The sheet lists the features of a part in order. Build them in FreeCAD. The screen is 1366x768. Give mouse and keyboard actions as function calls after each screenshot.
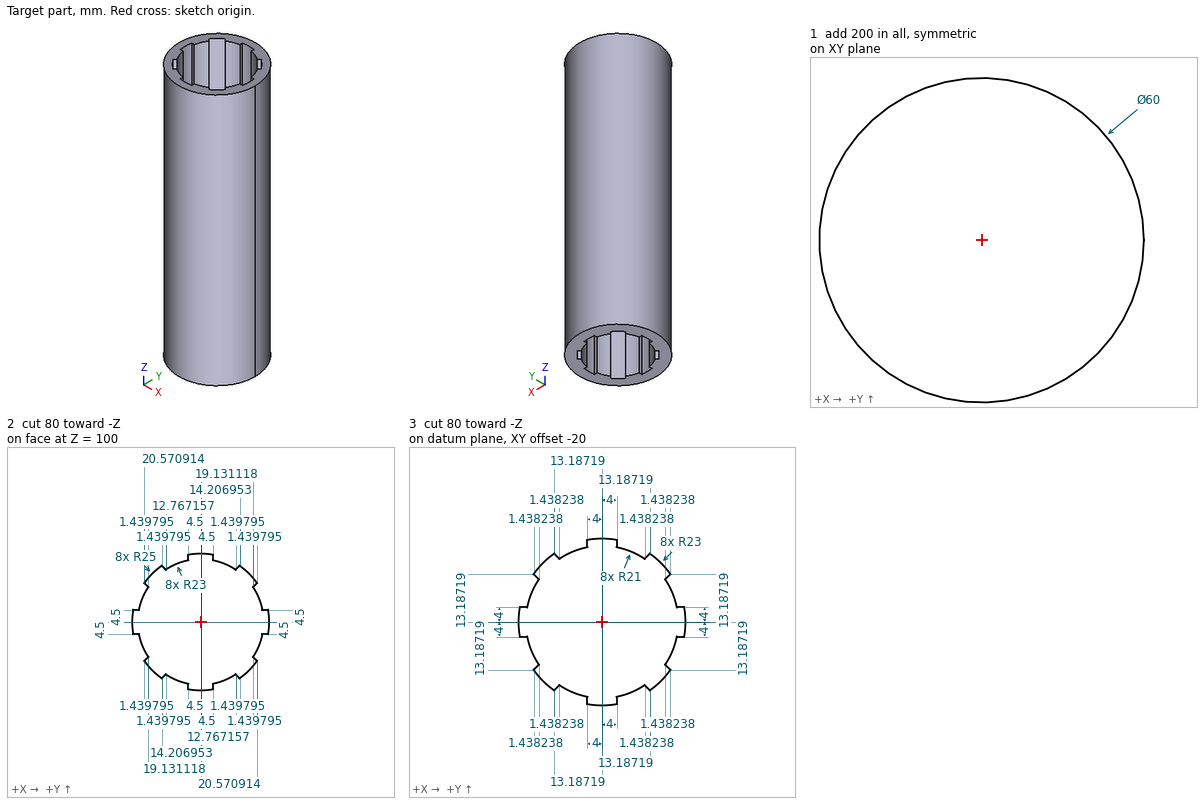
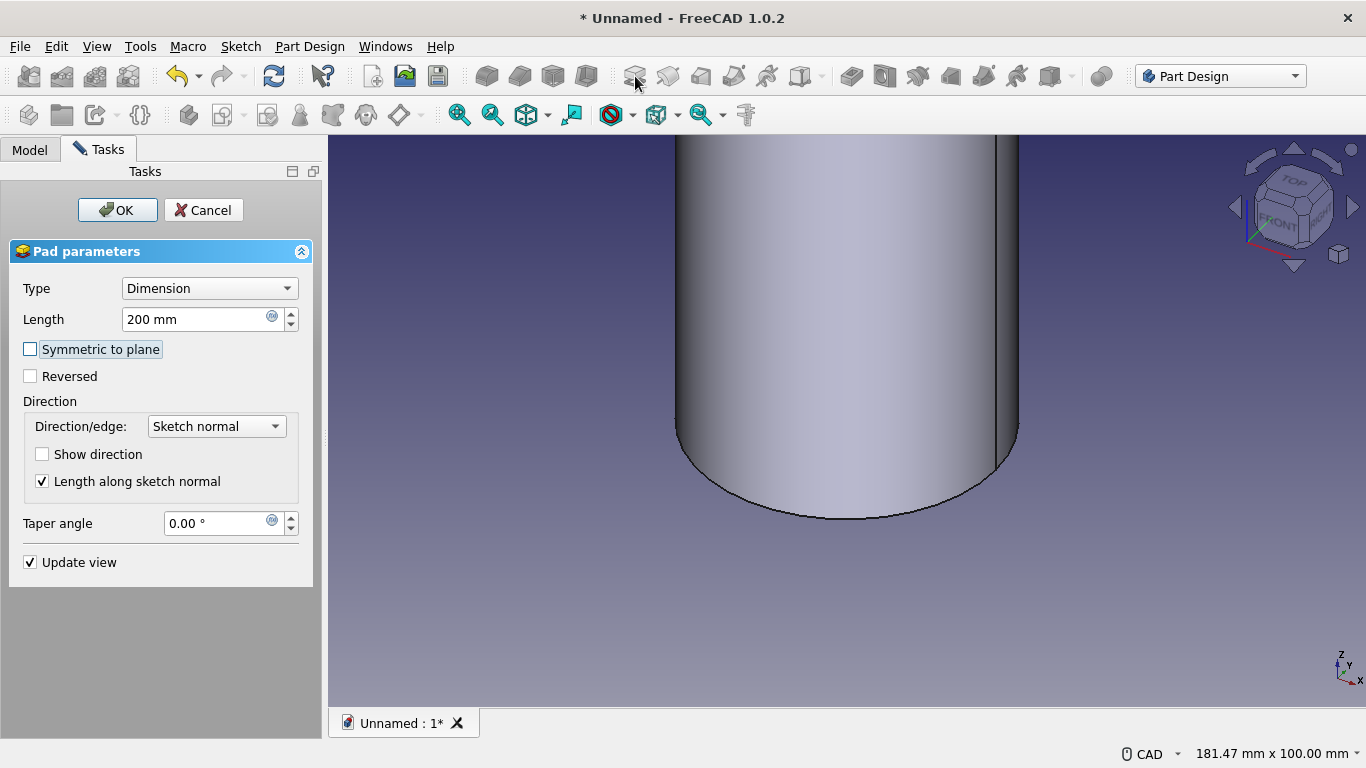
click(31, 349)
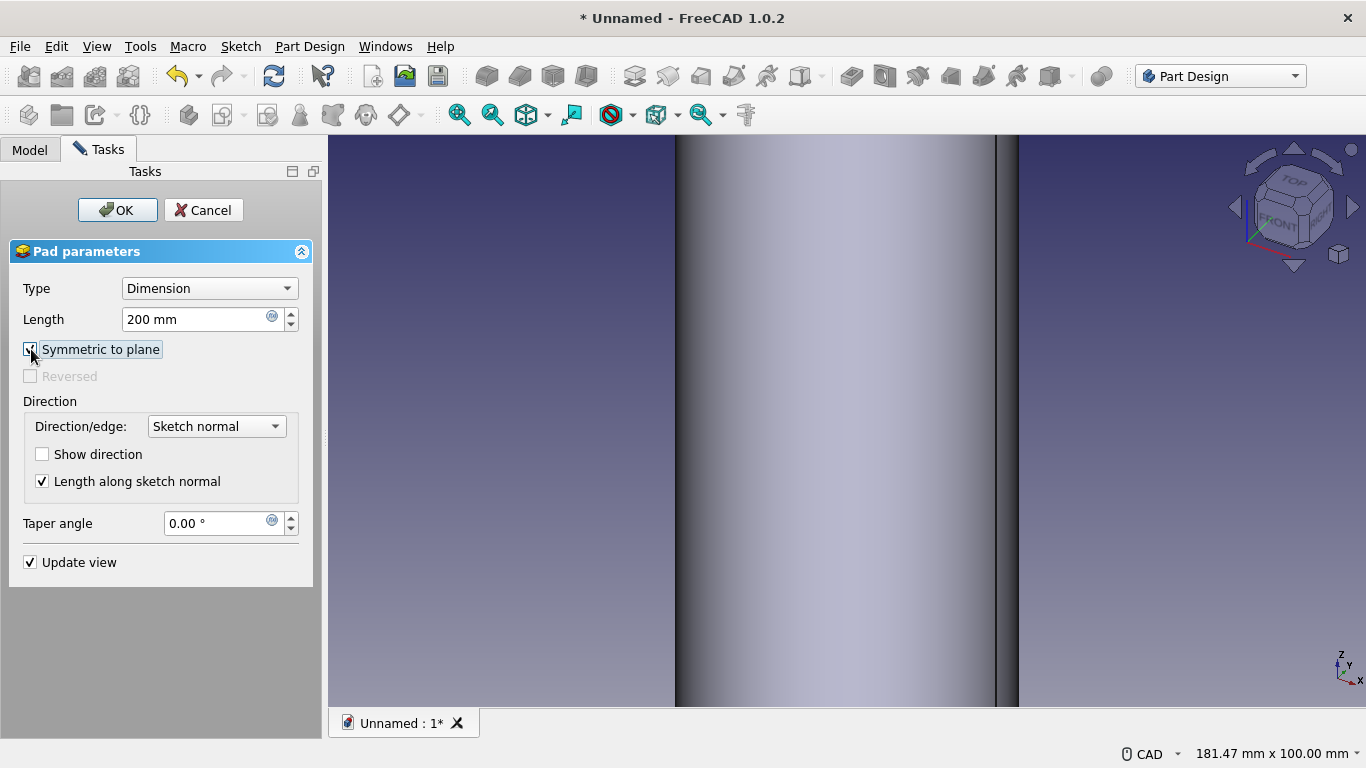
click(118, 210)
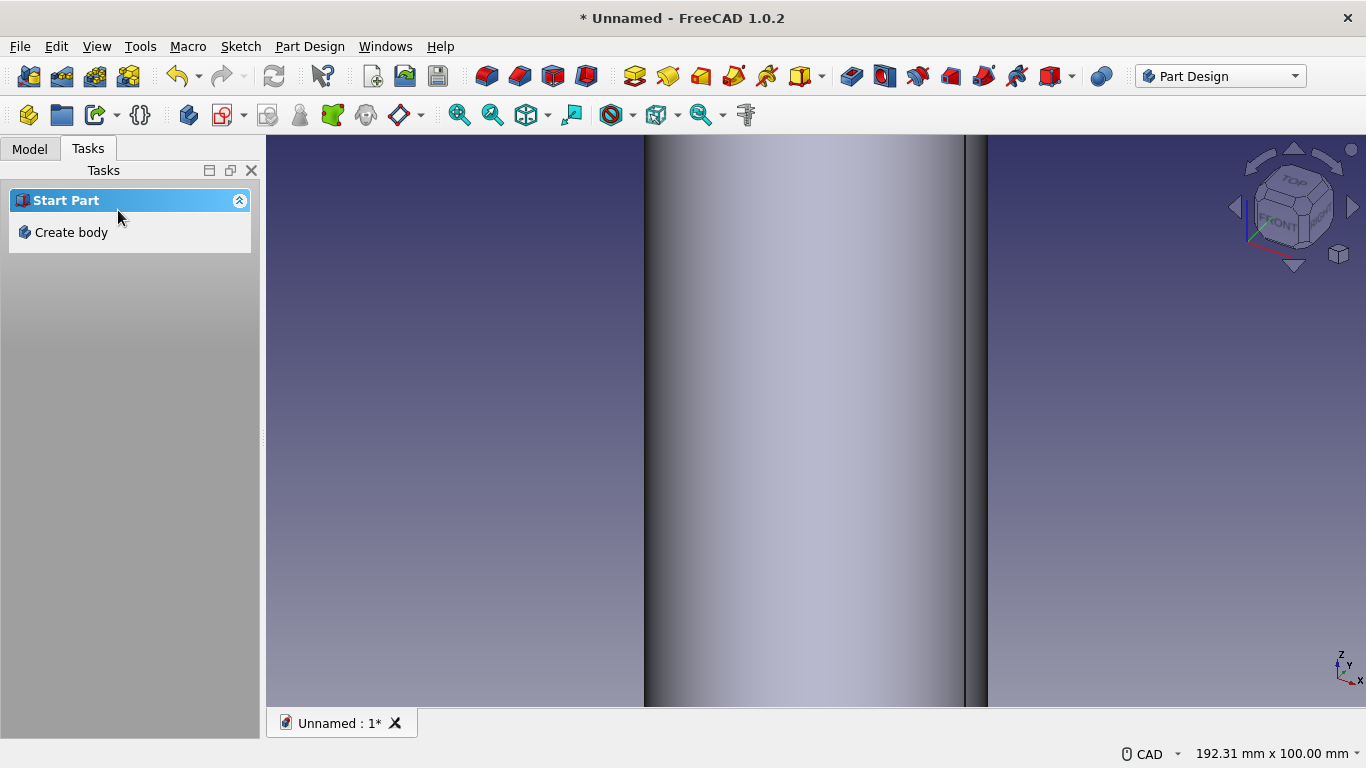
click(460, 116)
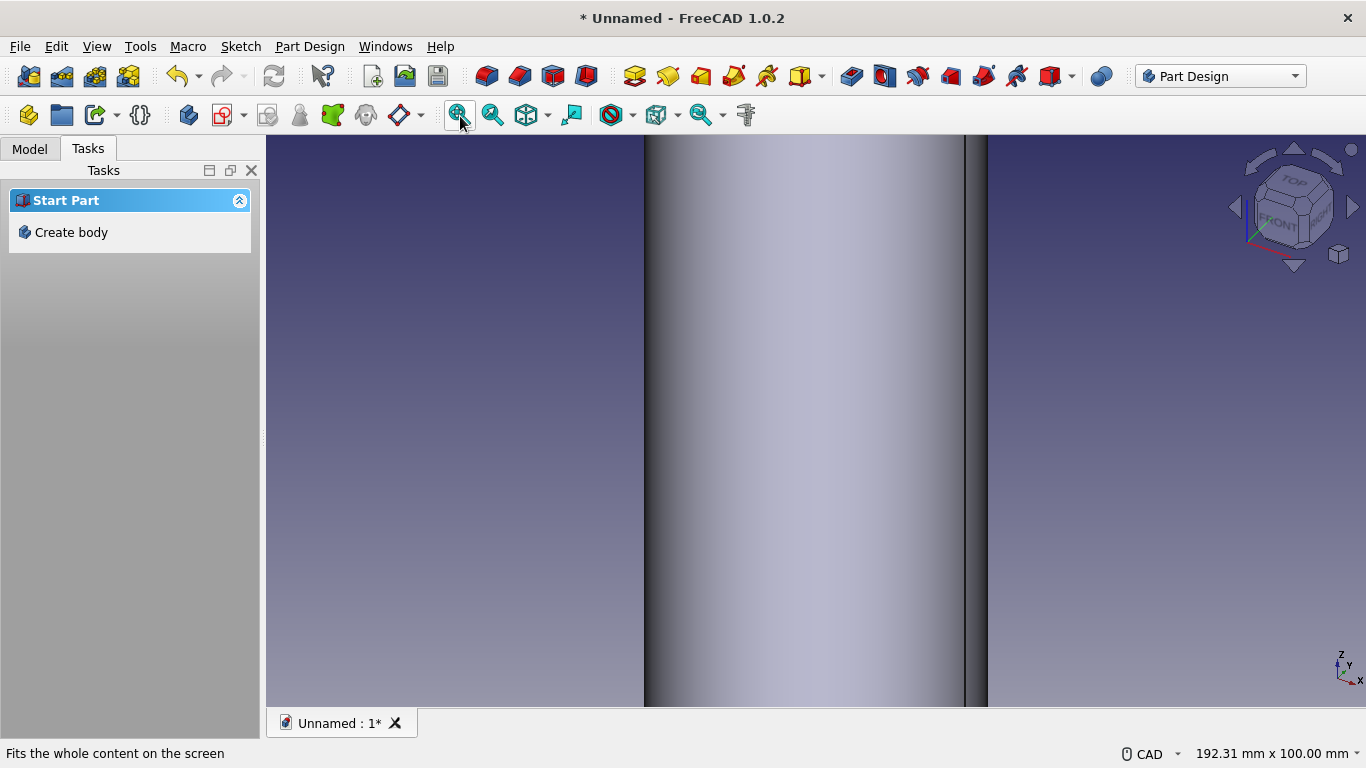
click(816, 204)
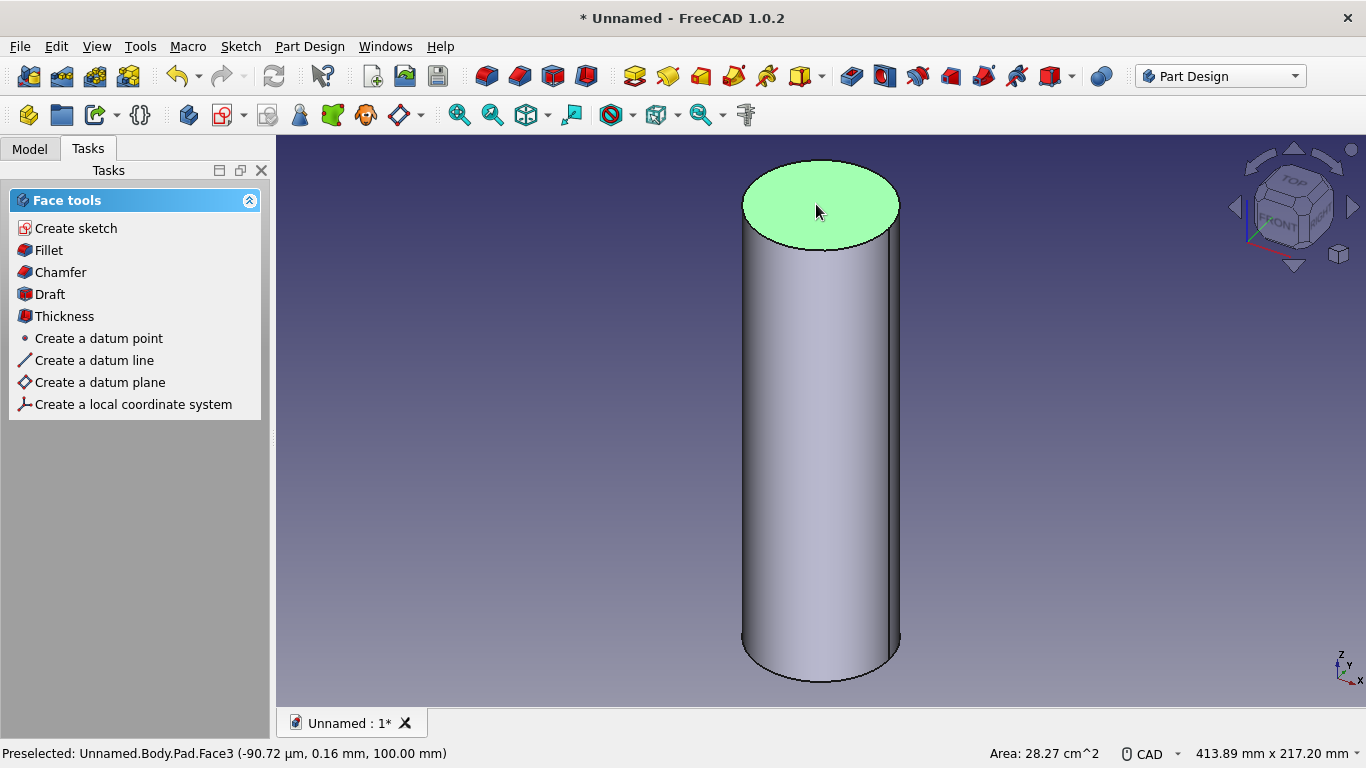
click(222, 116)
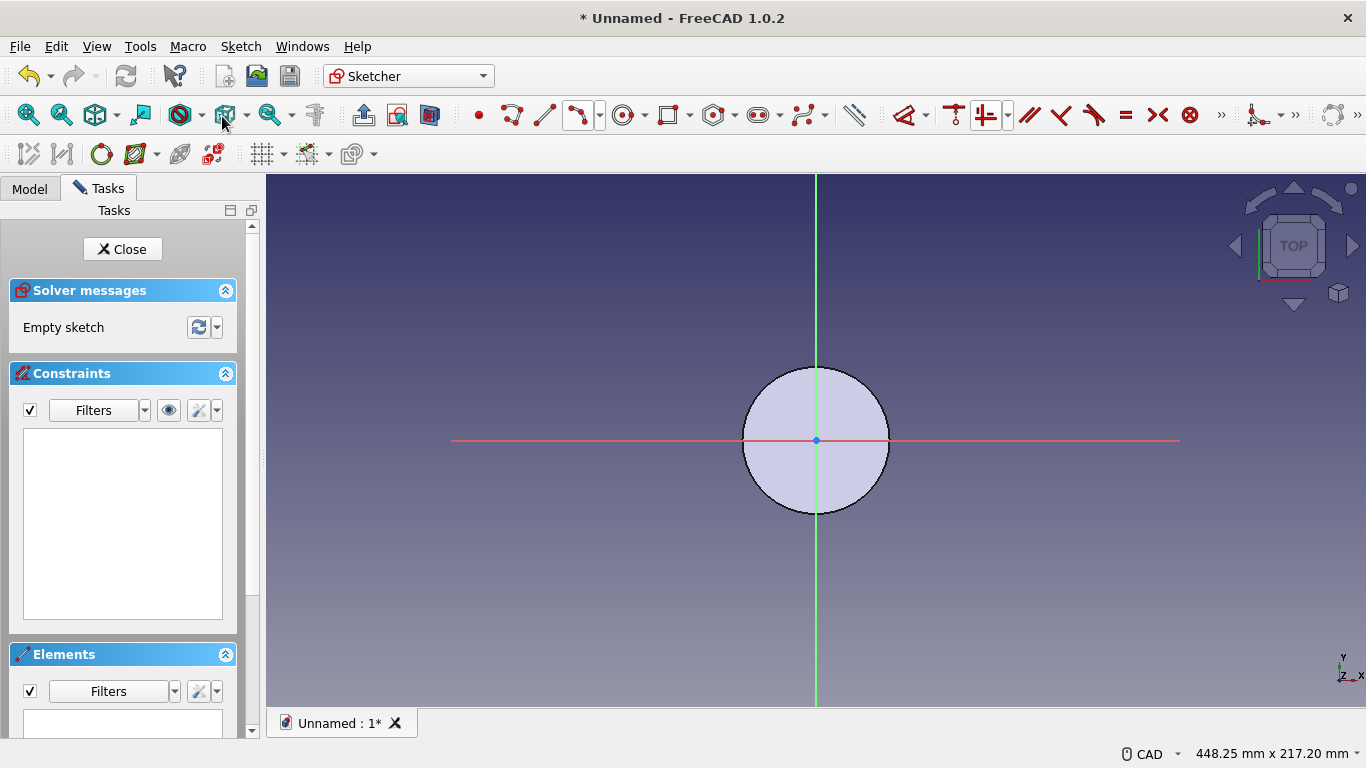
scroll(856, 440, up, 5)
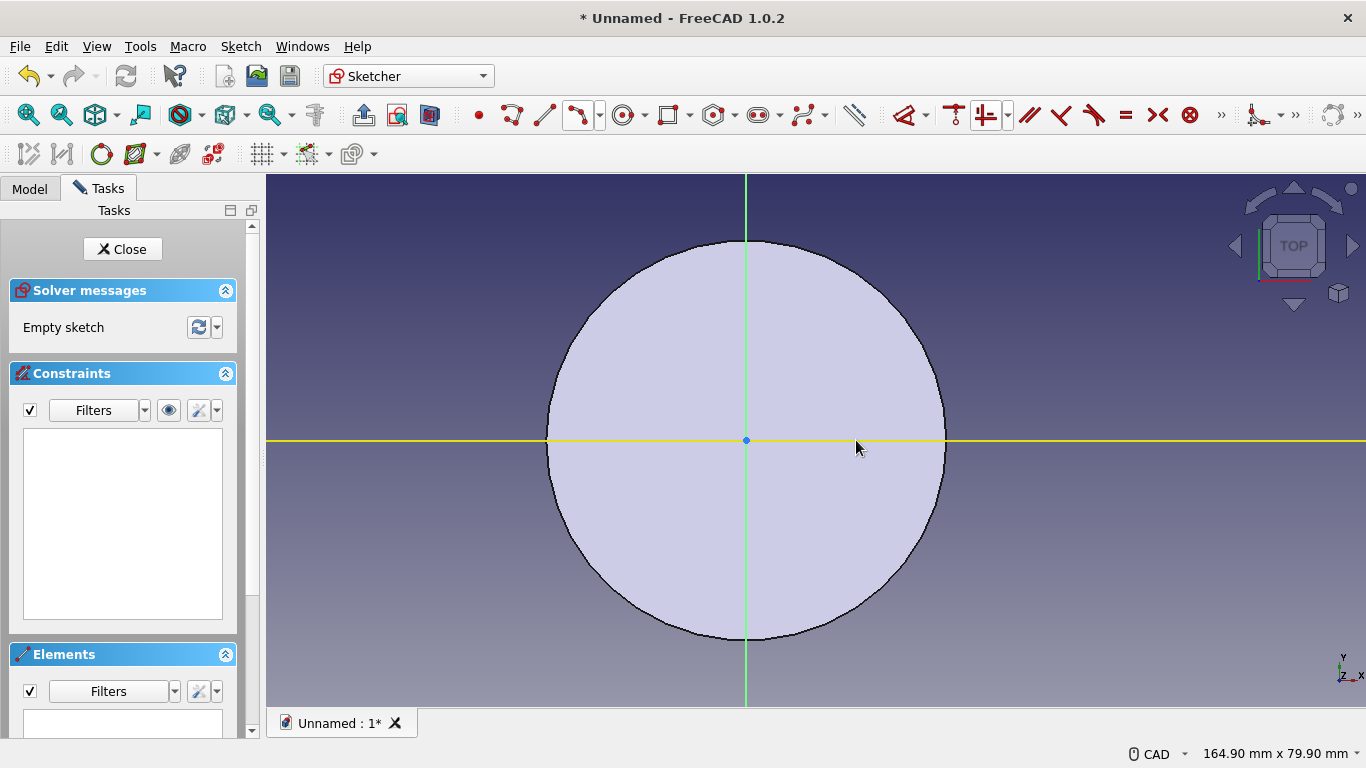
click(545, 116)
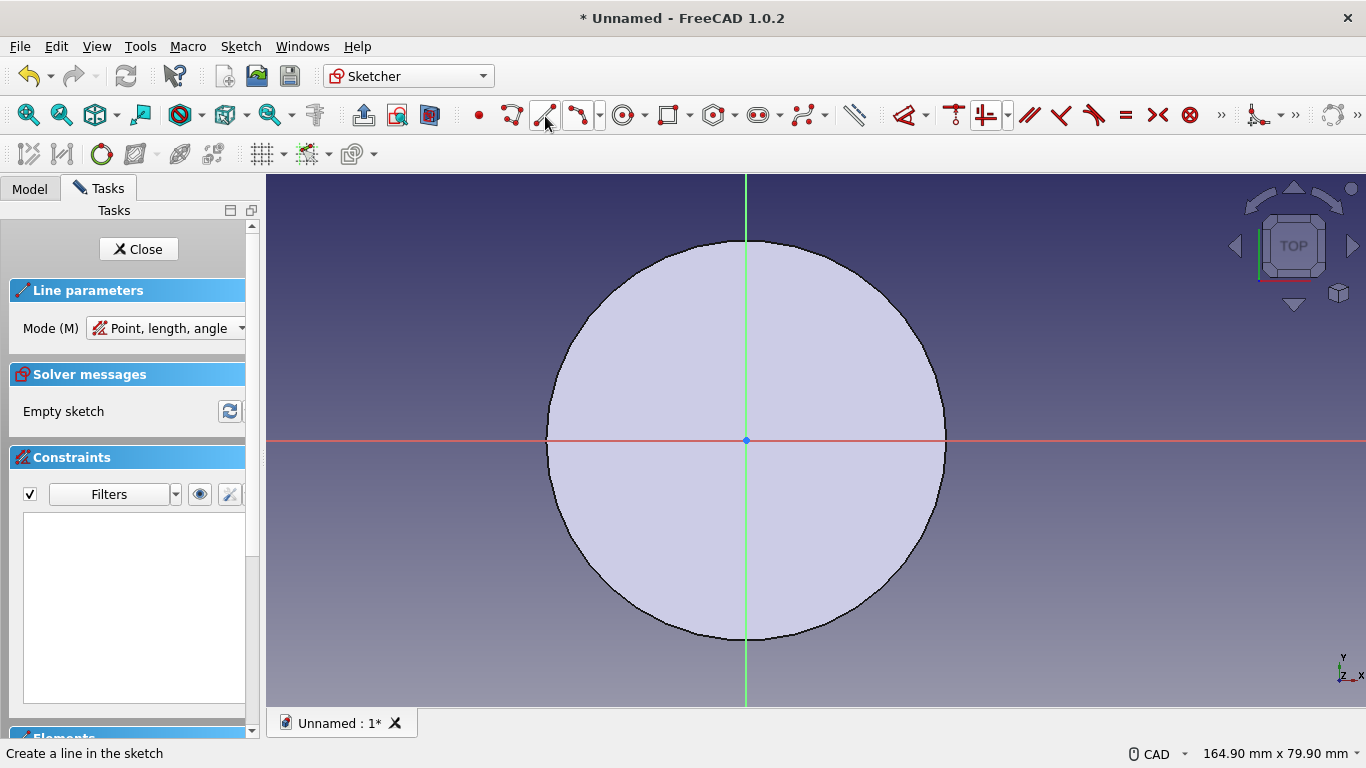
click(716, 276)
click(716, 290)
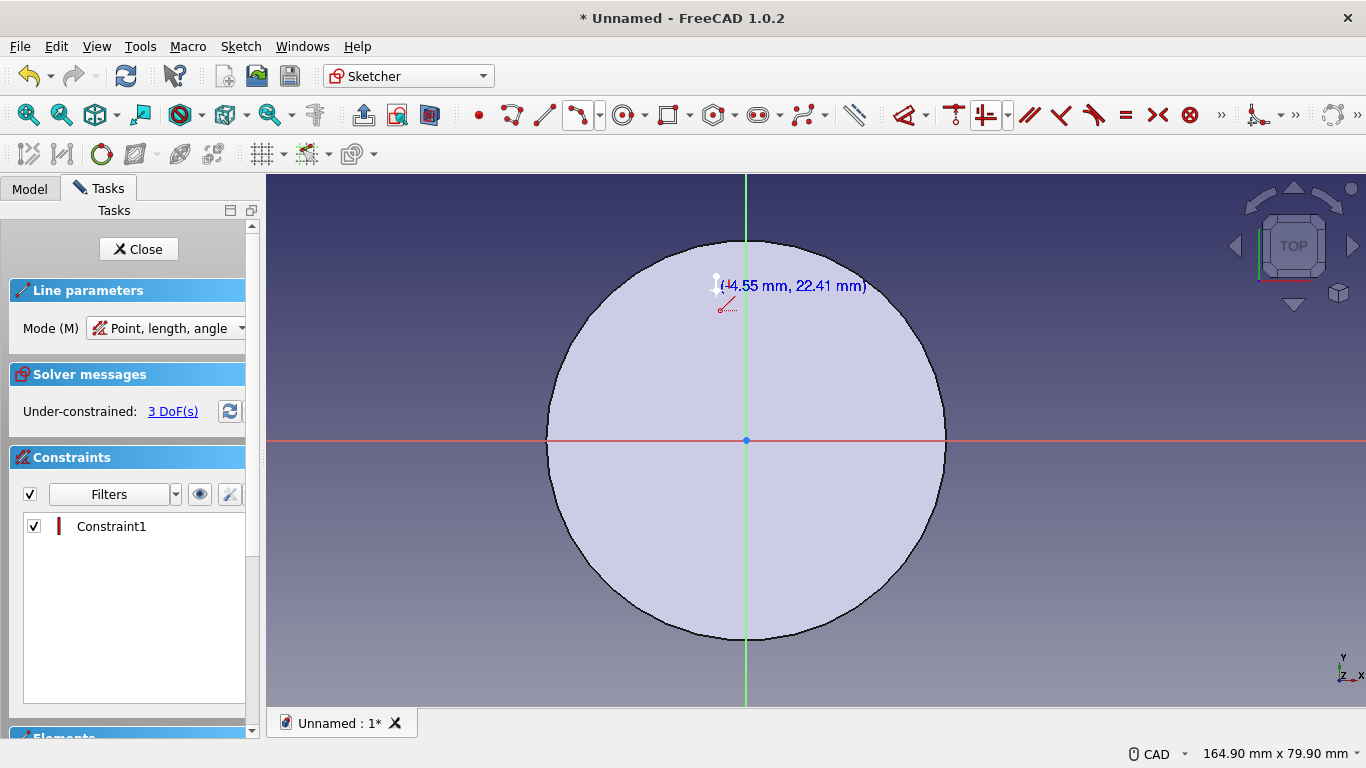
click(661, 313)
click(652, 303)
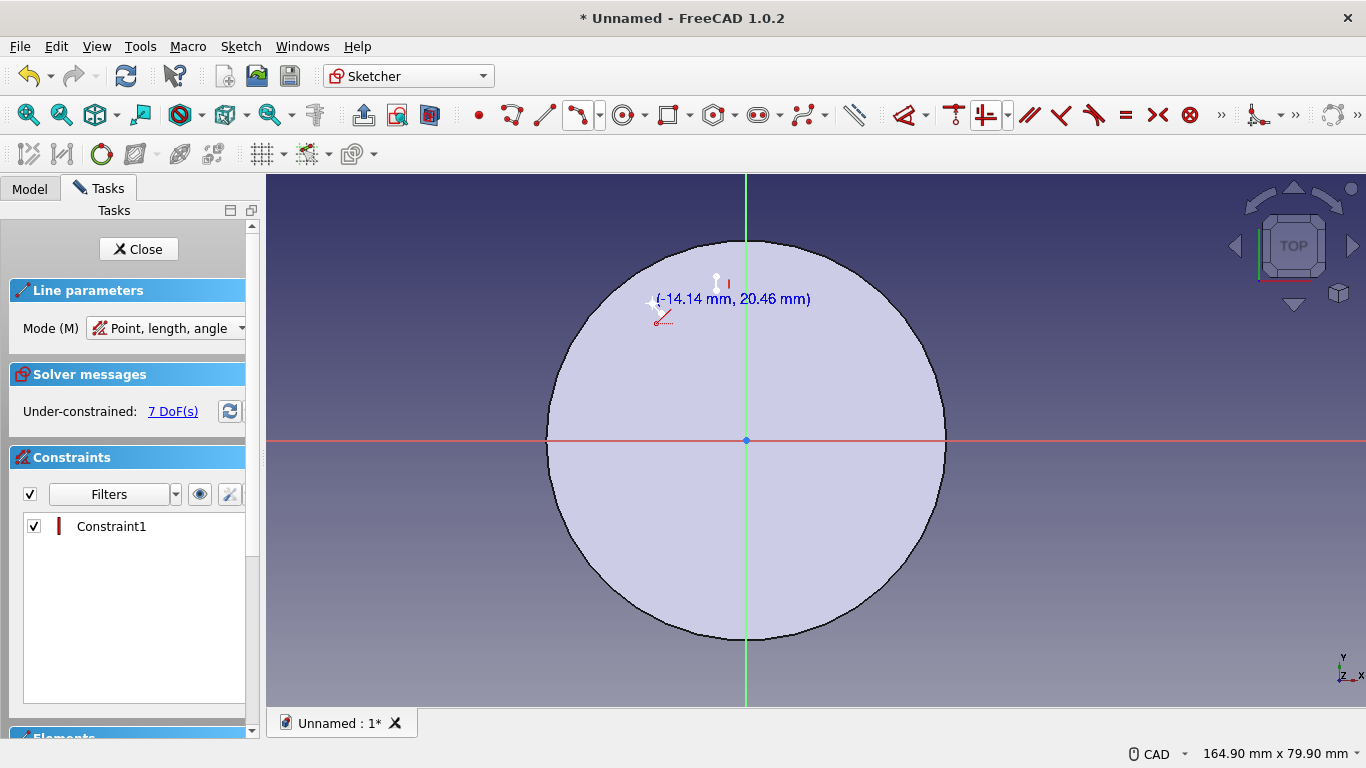
click(609, 346)
click(619, 355)